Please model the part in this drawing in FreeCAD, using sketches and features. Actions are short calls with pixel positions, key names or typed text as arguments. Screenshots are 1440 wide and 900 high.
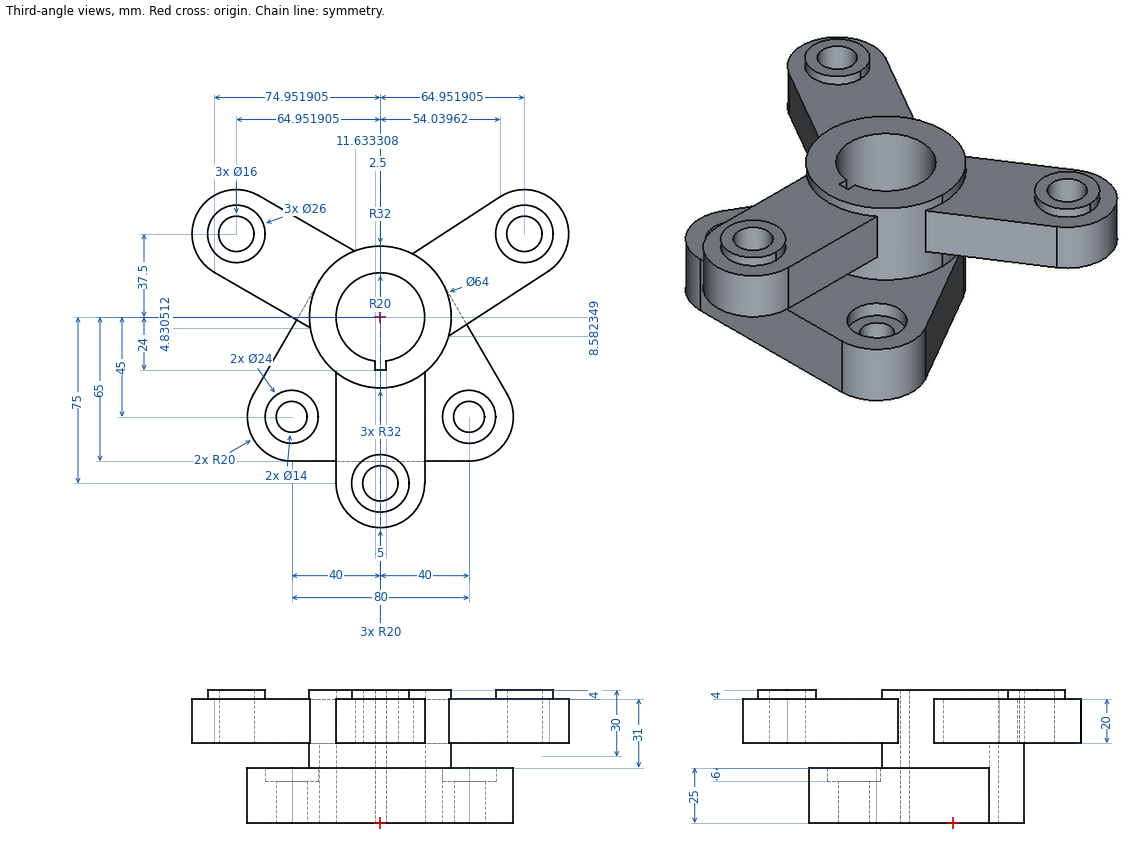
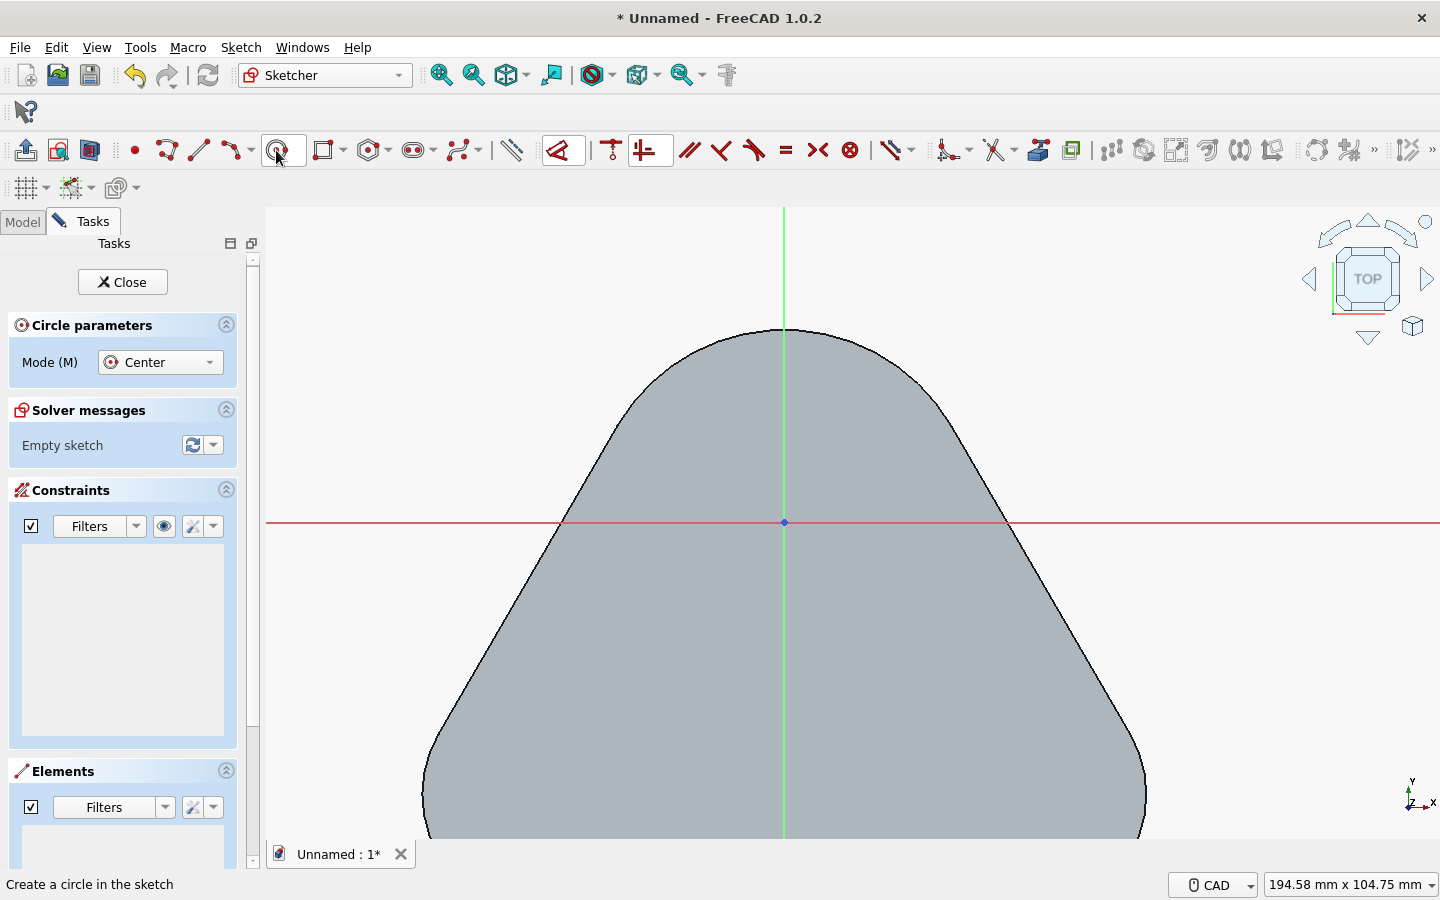
click(784, 523)
move(921, 386)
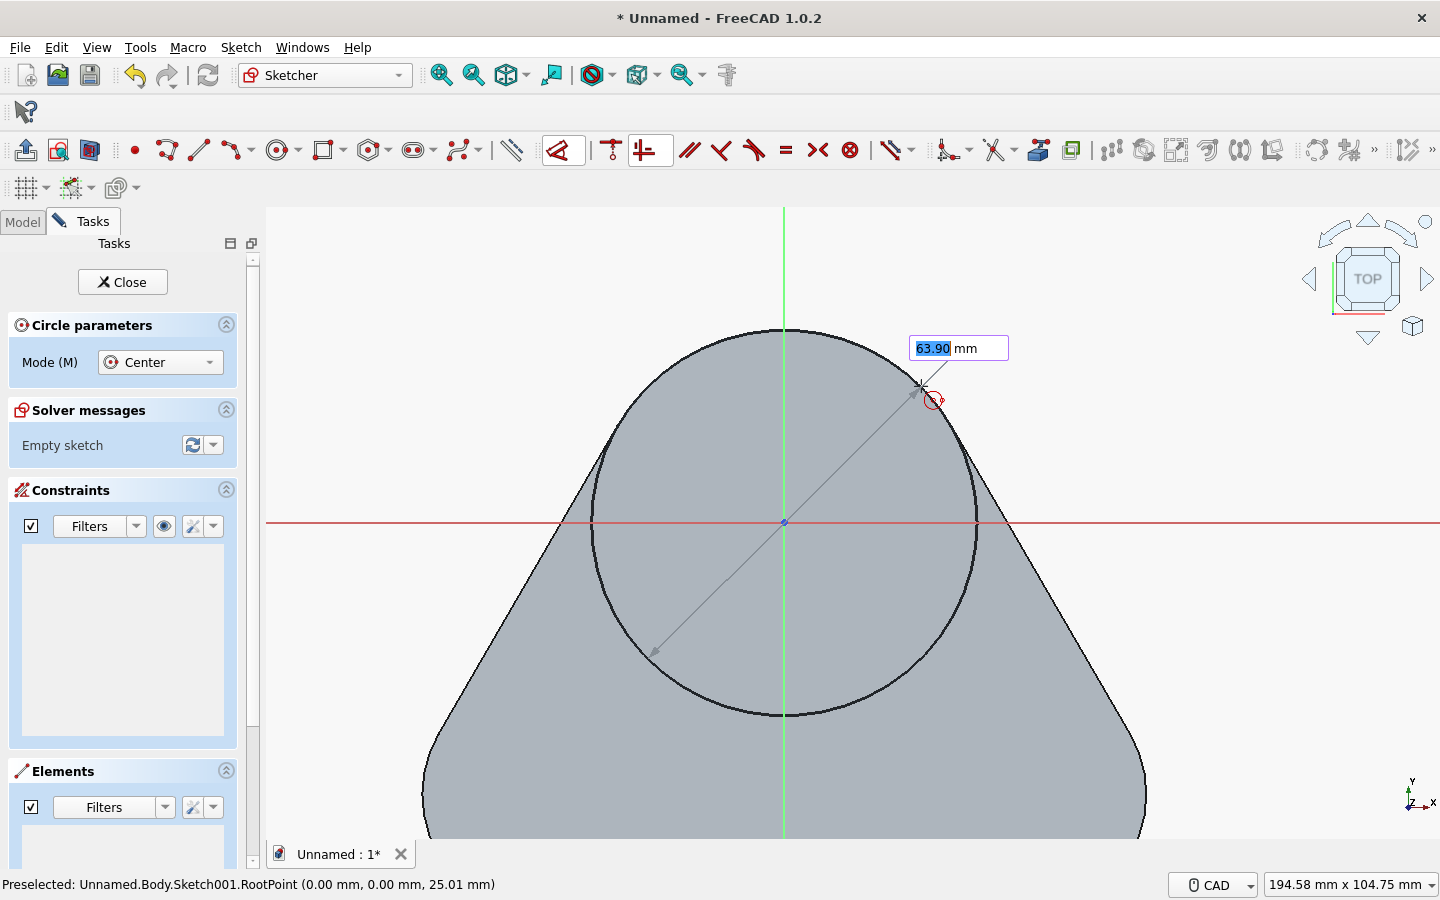
text(64)
key(Return)
key(Escape)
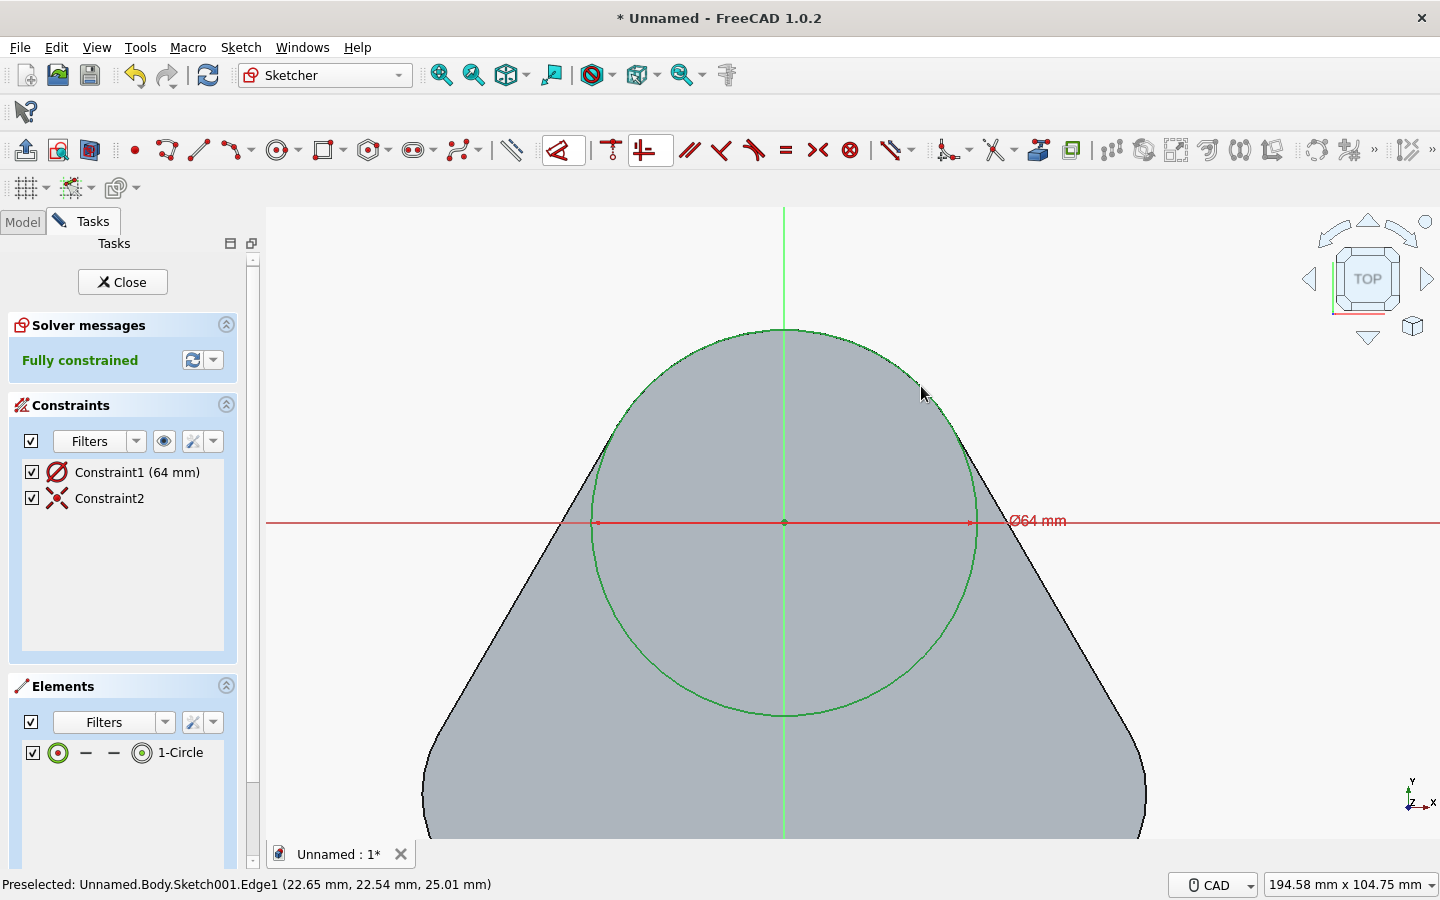
click(123, 282)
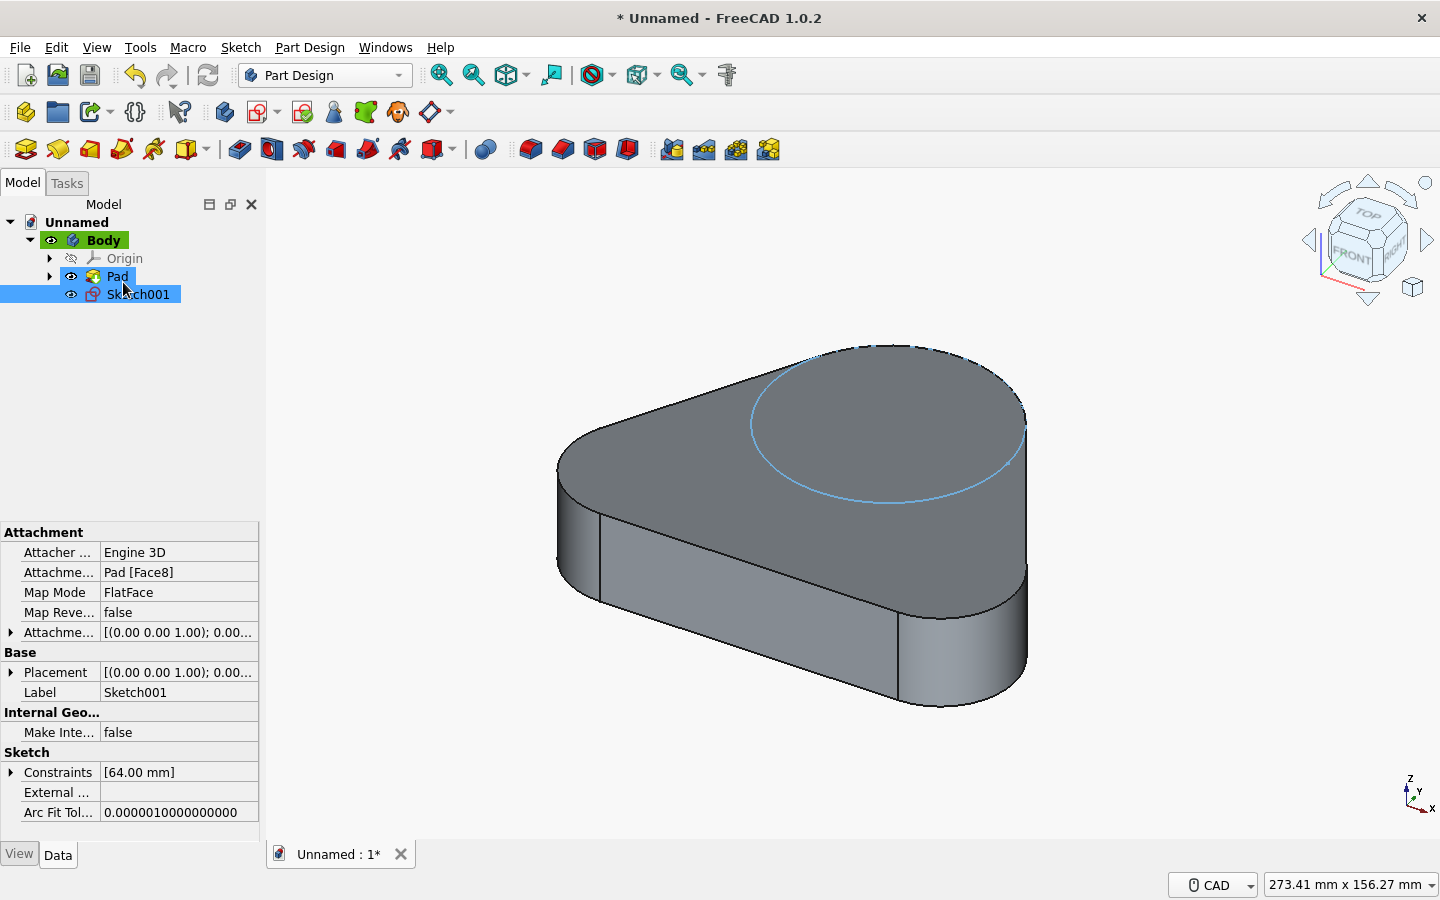
click(26, 150)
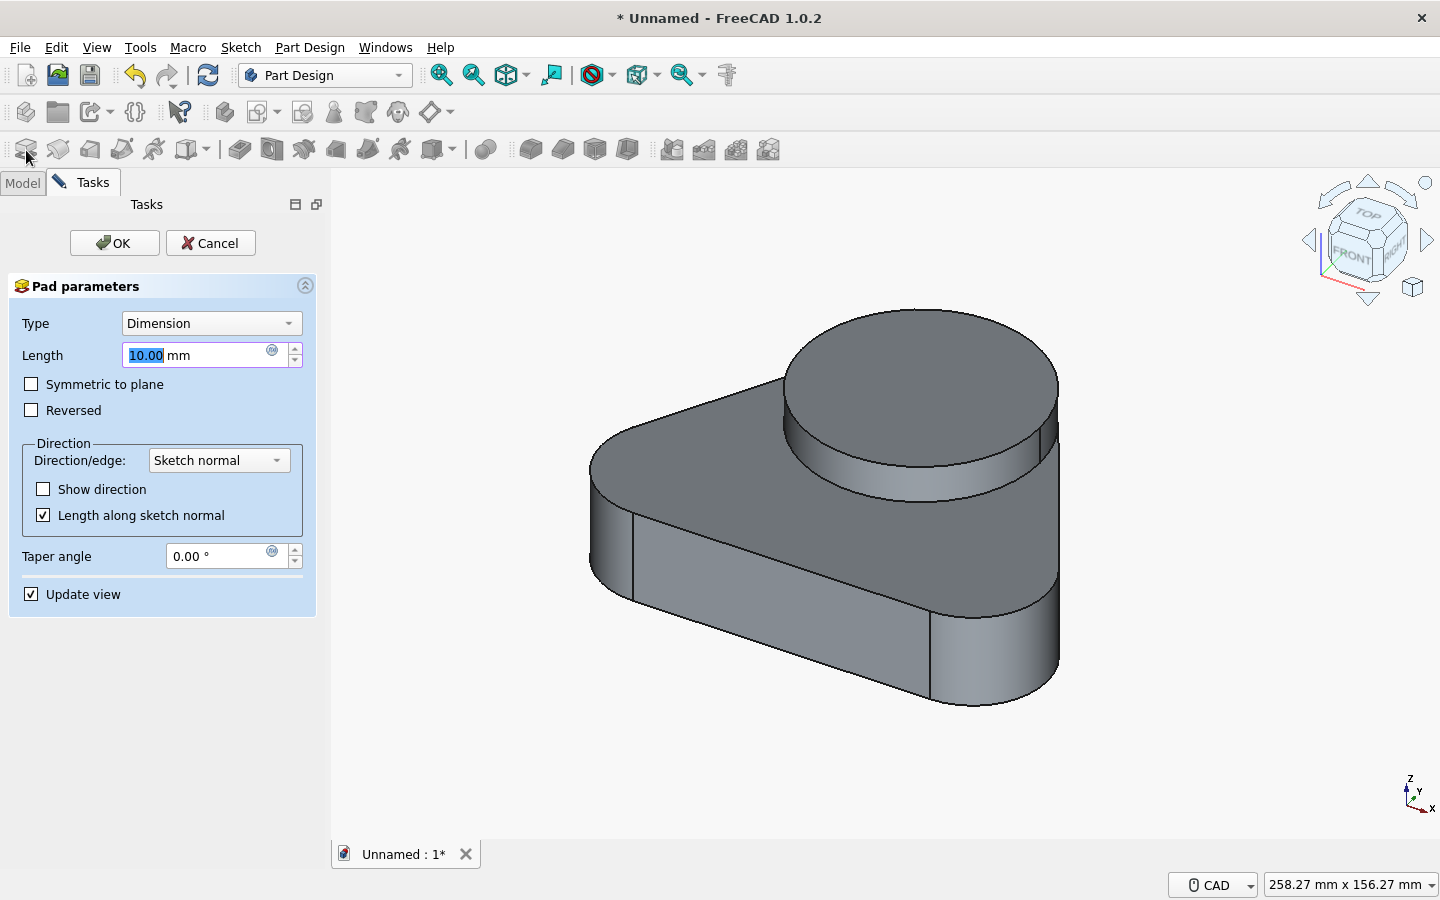
text(31)
key(Tab)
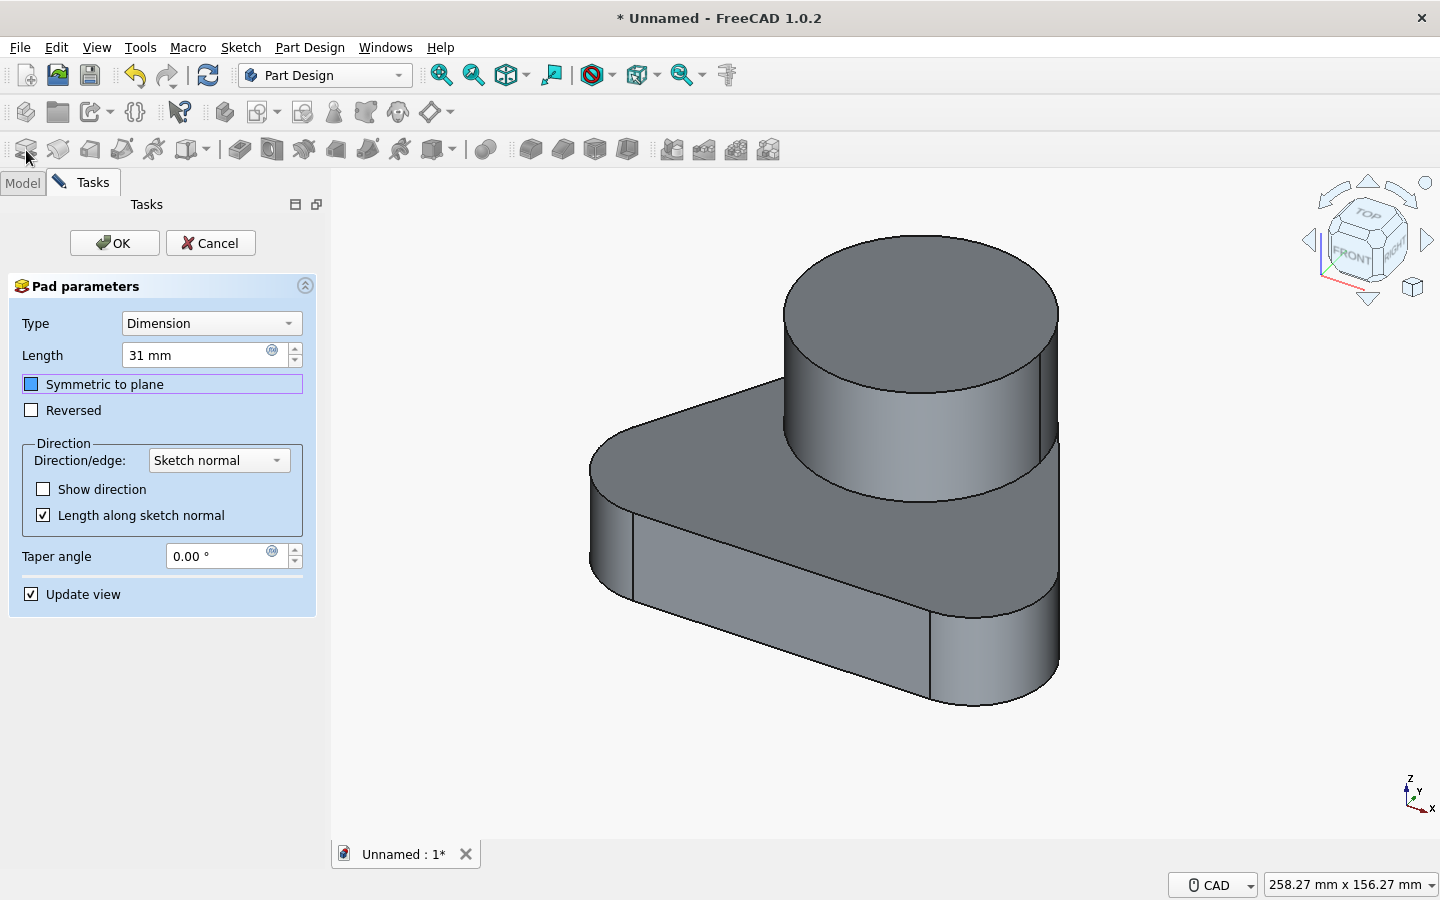
click(115, 243)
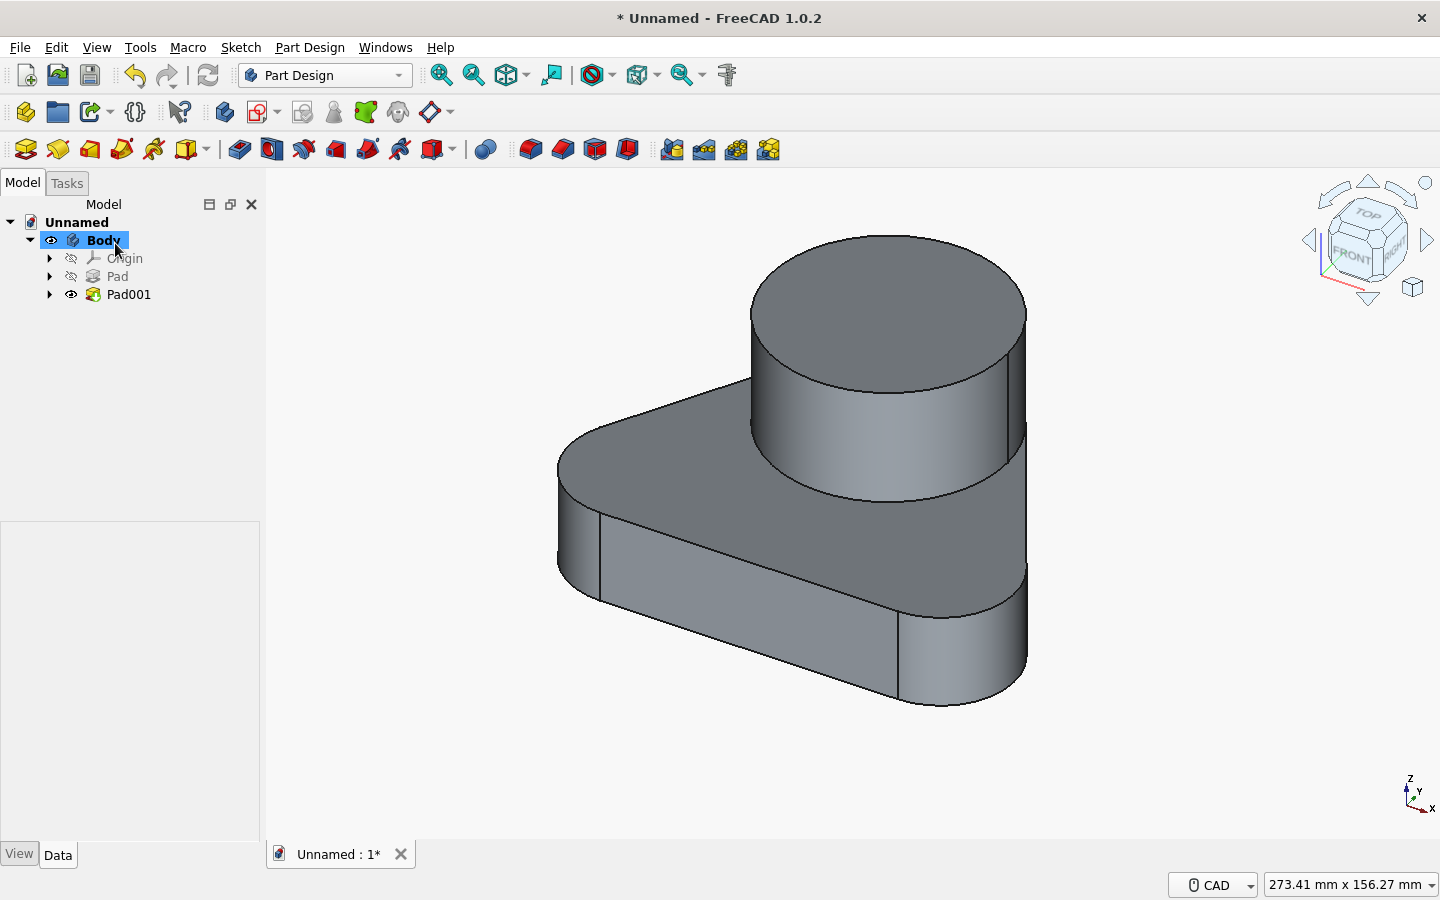
click(50, 258)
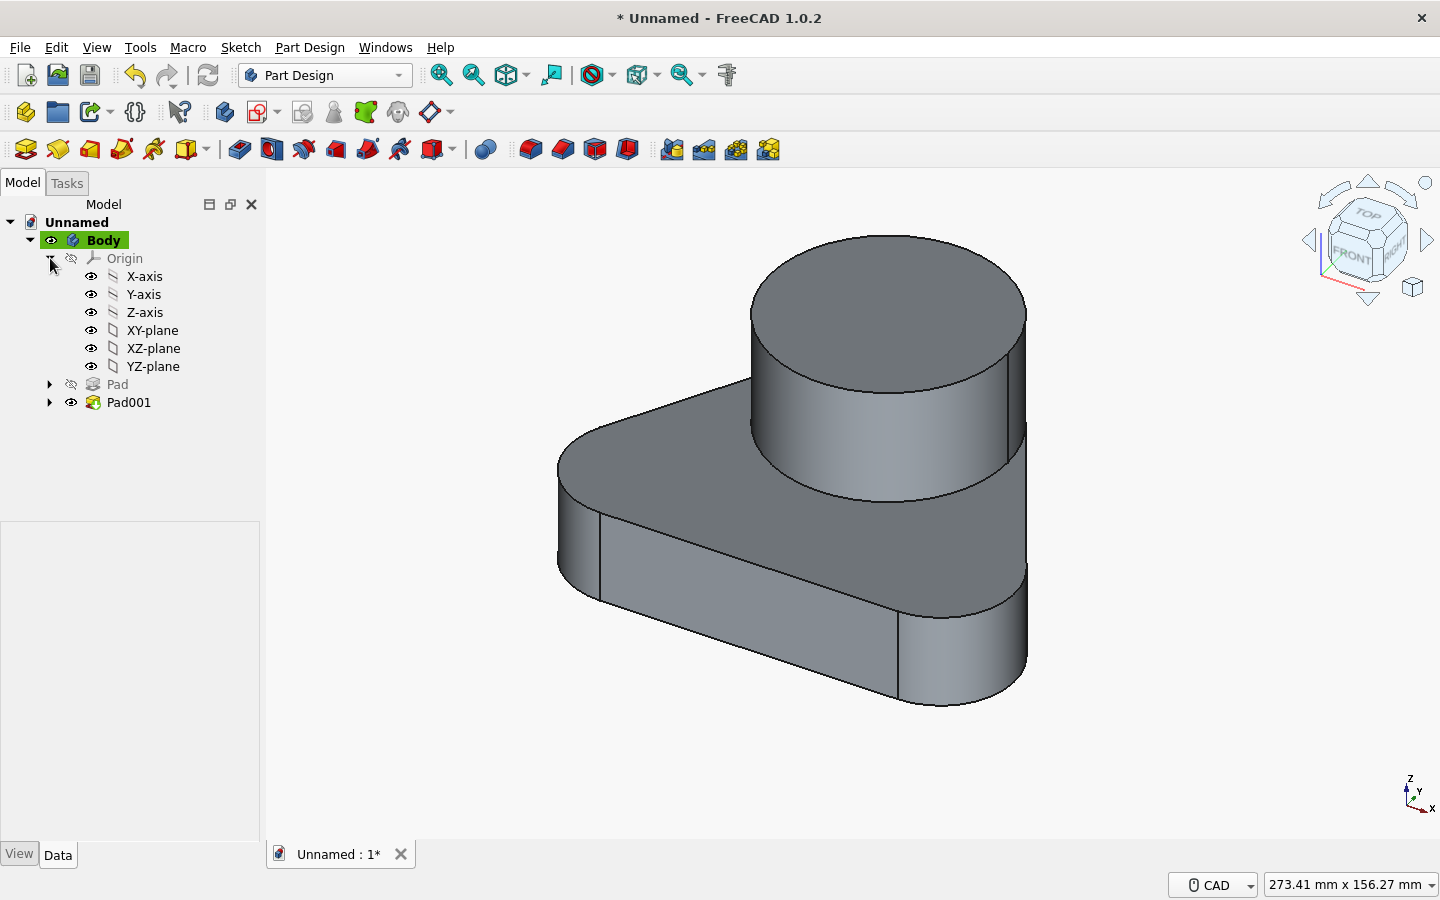
click(136, 330)